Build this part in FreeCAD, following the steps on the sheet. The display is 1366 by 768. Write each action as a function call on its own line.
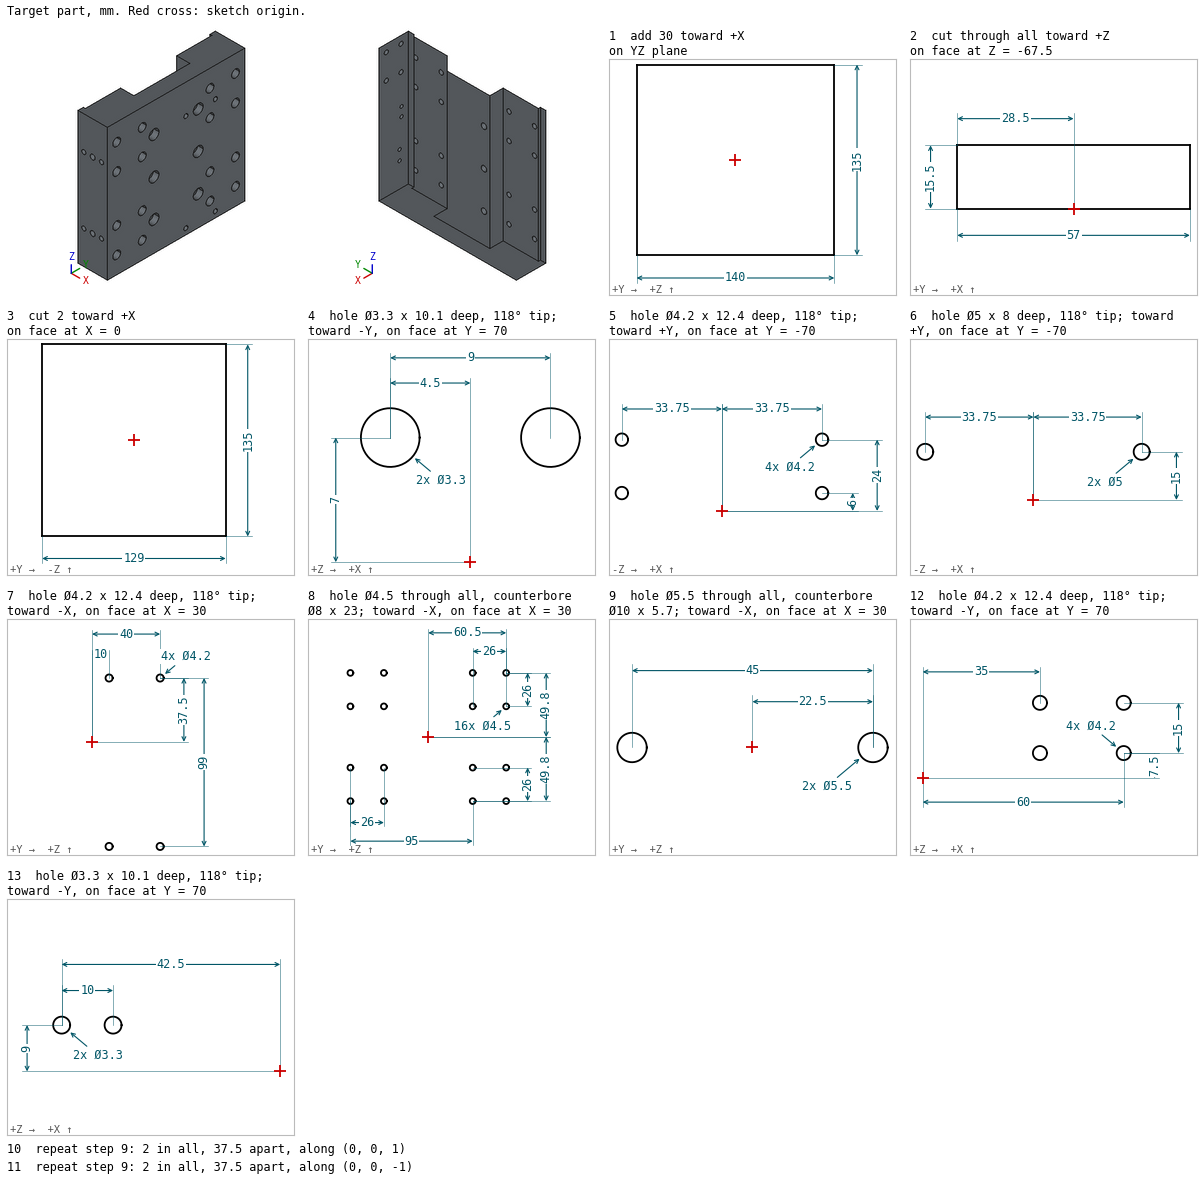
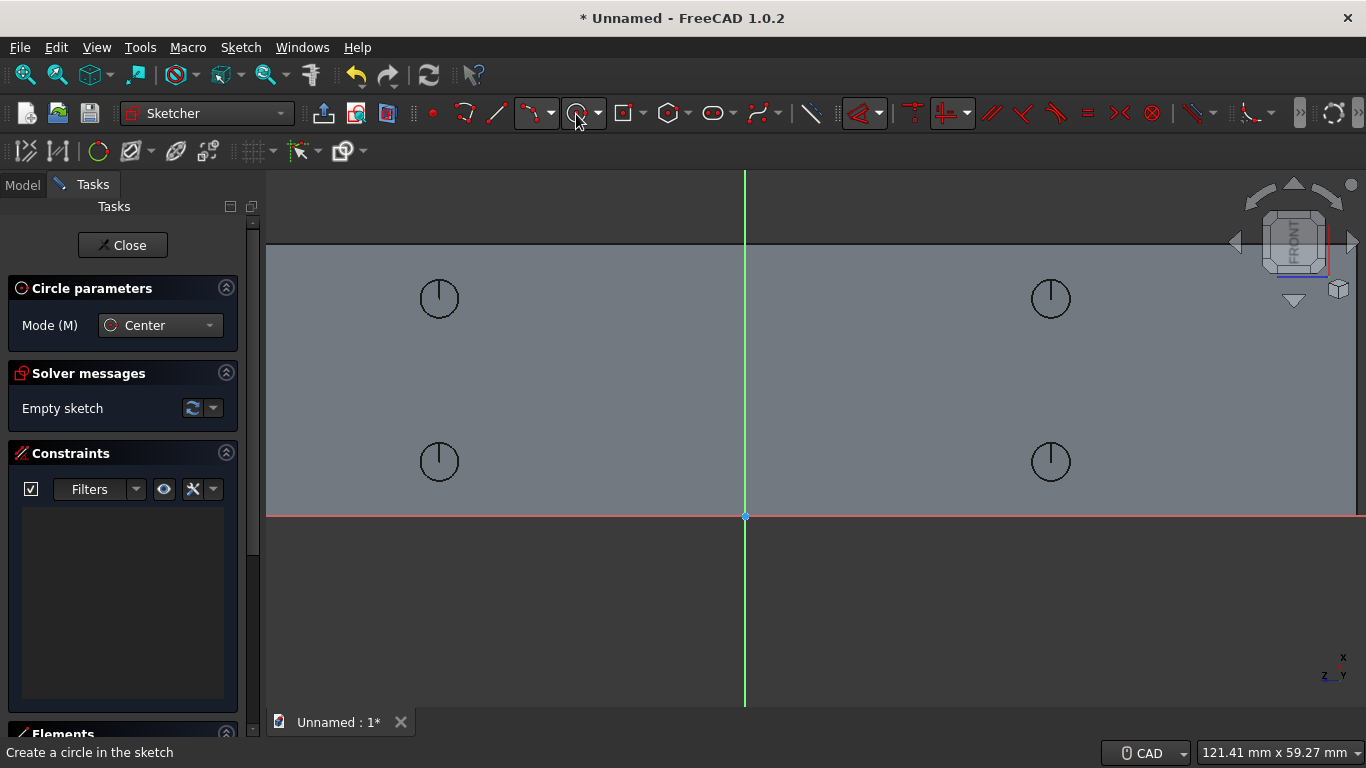
click(1051, 380)
click(1067, 364)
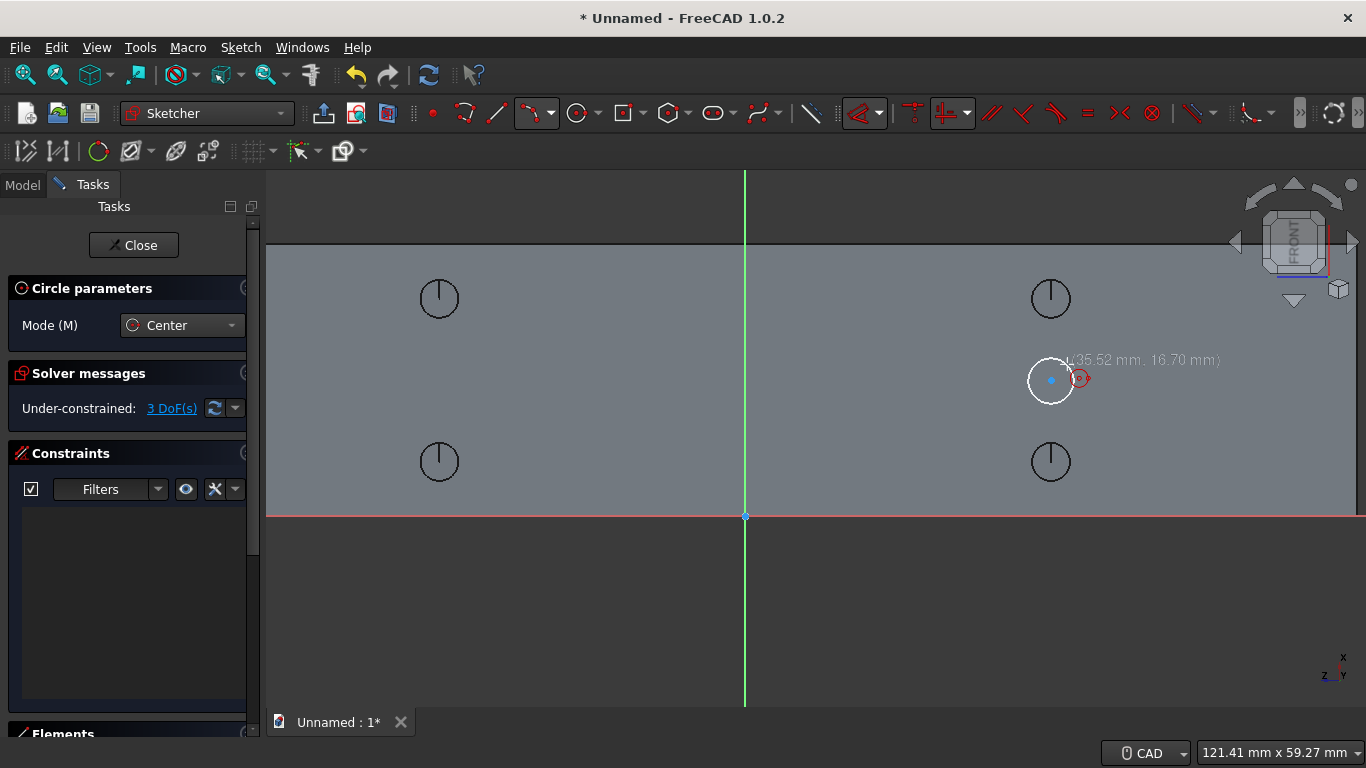
click(439, 380)
click(455, 364)
key(Escape)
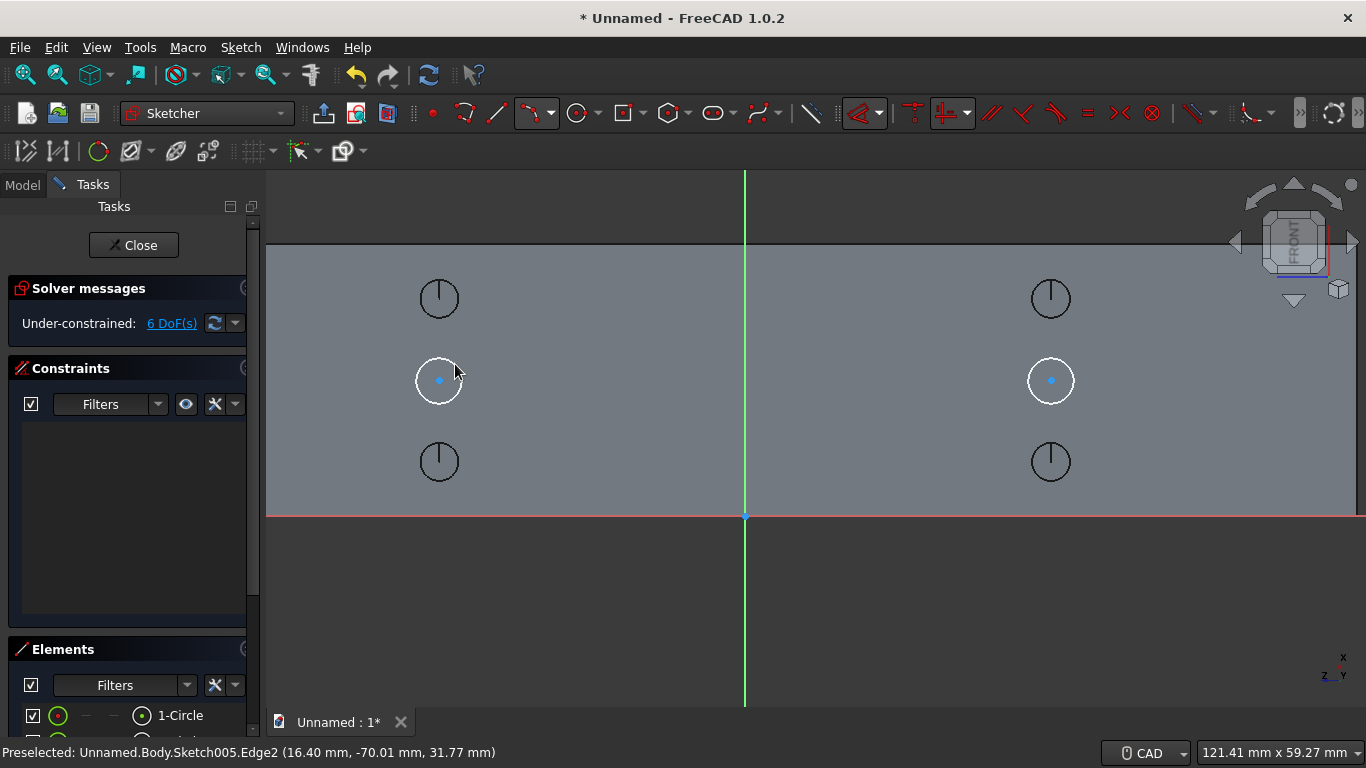
click(1067, 365)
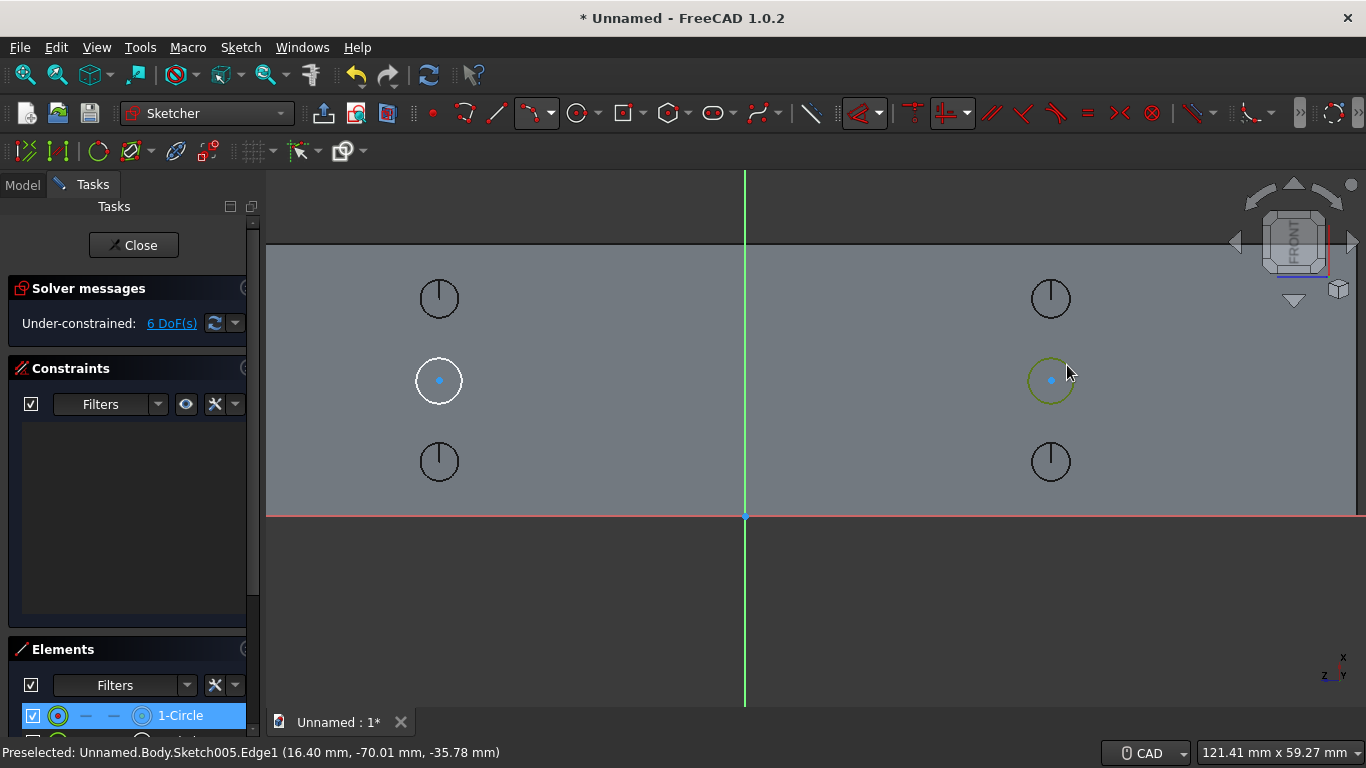
click(455, 365)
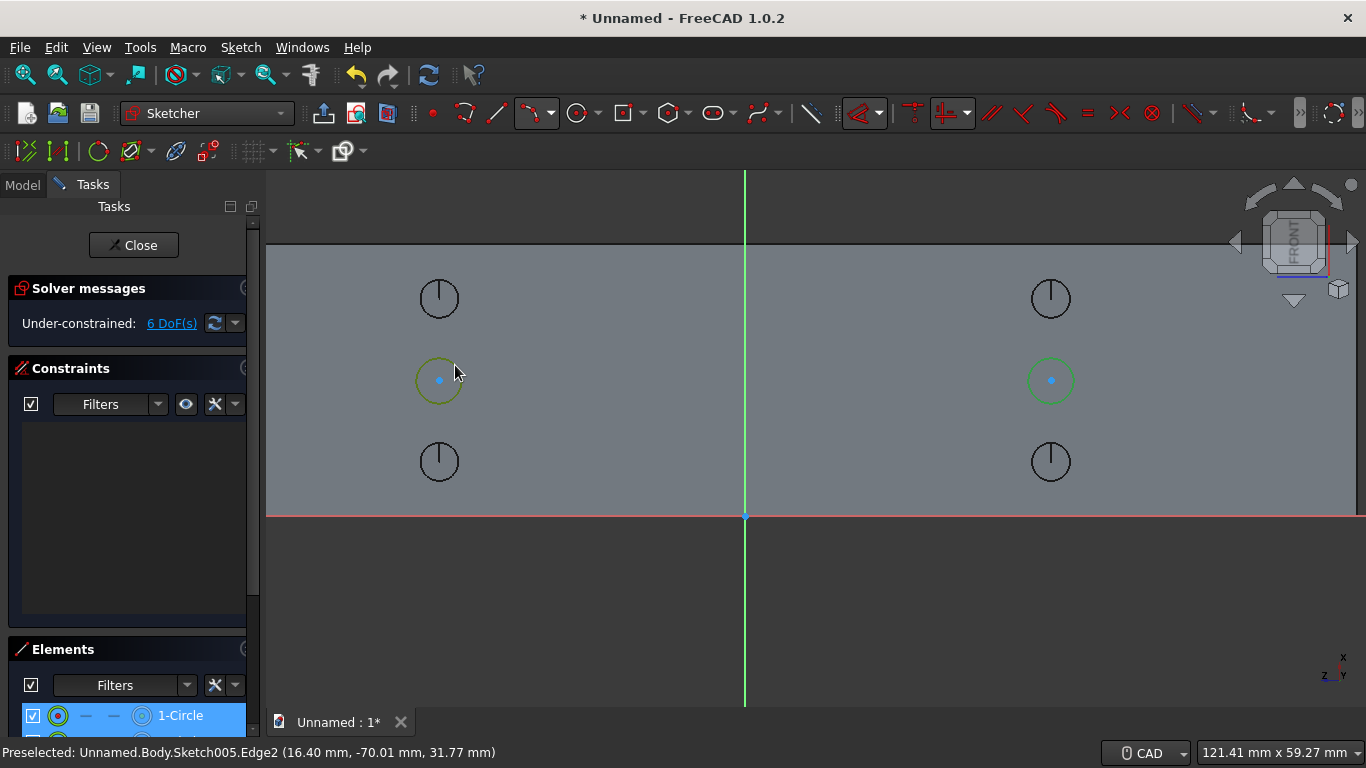
click(1088, 114)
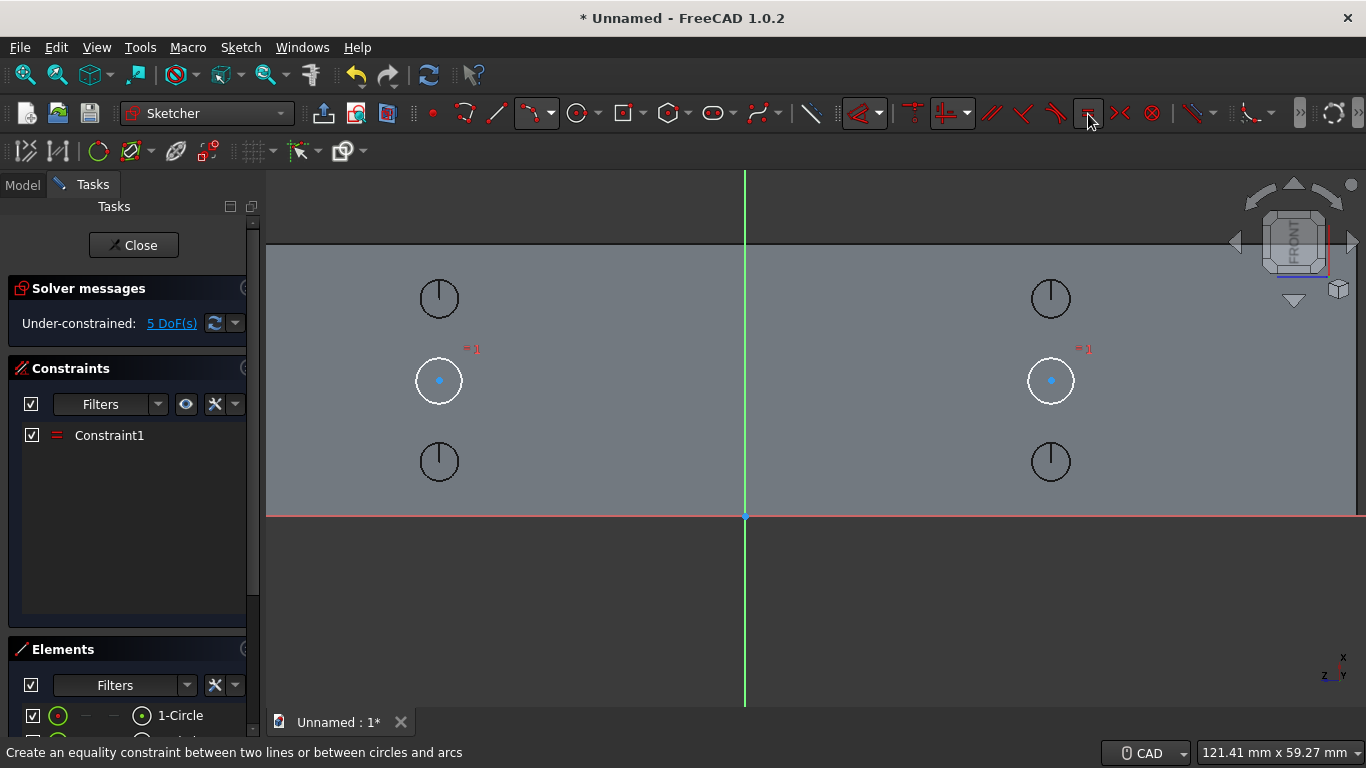
click(1051, 381)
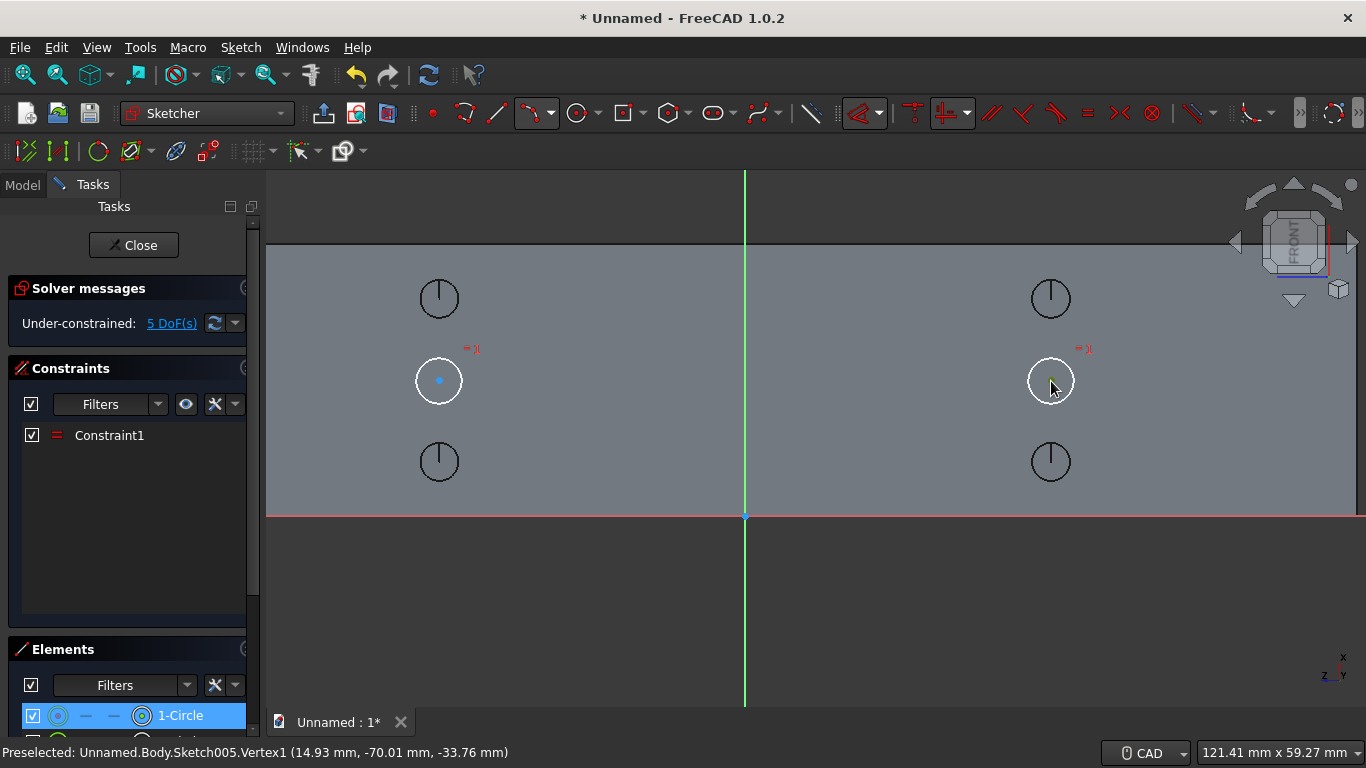
click(439, 381)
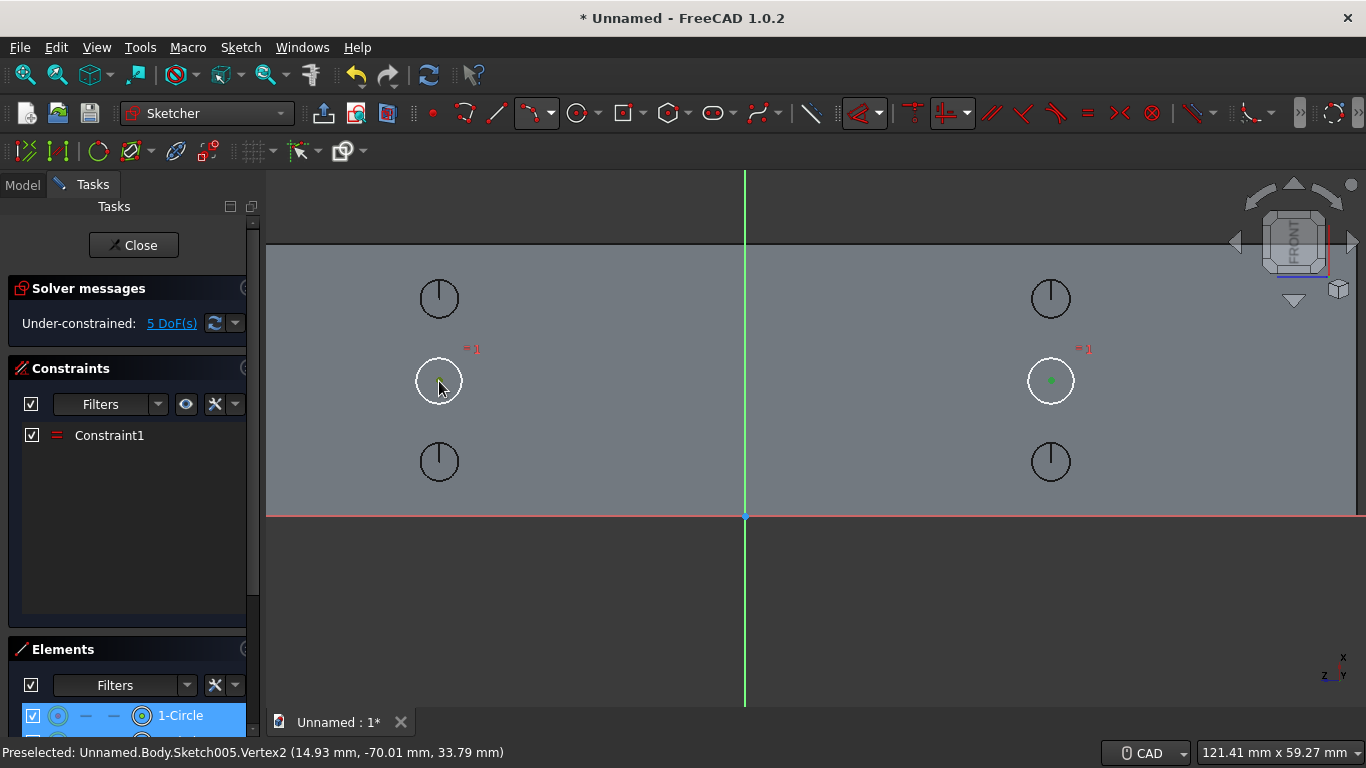
click(970, 114)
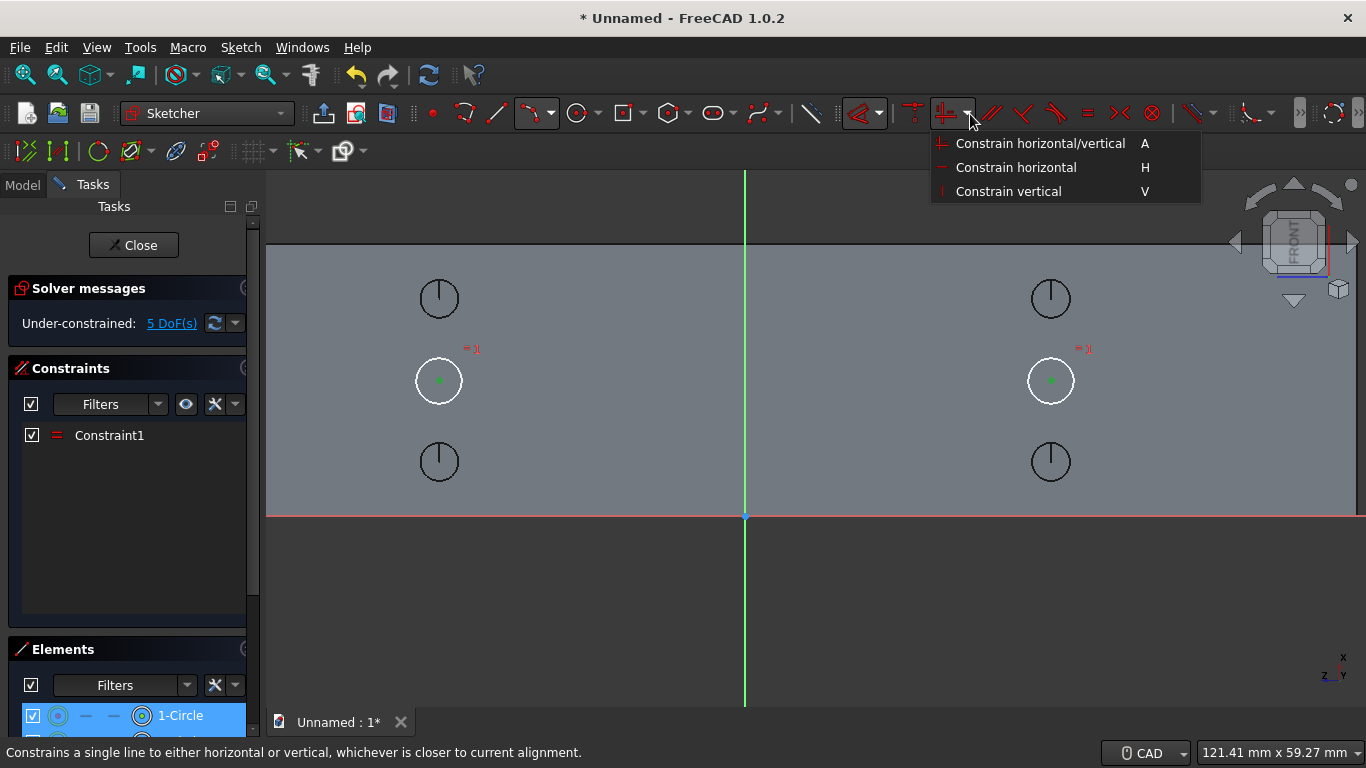
click(1066, 167)